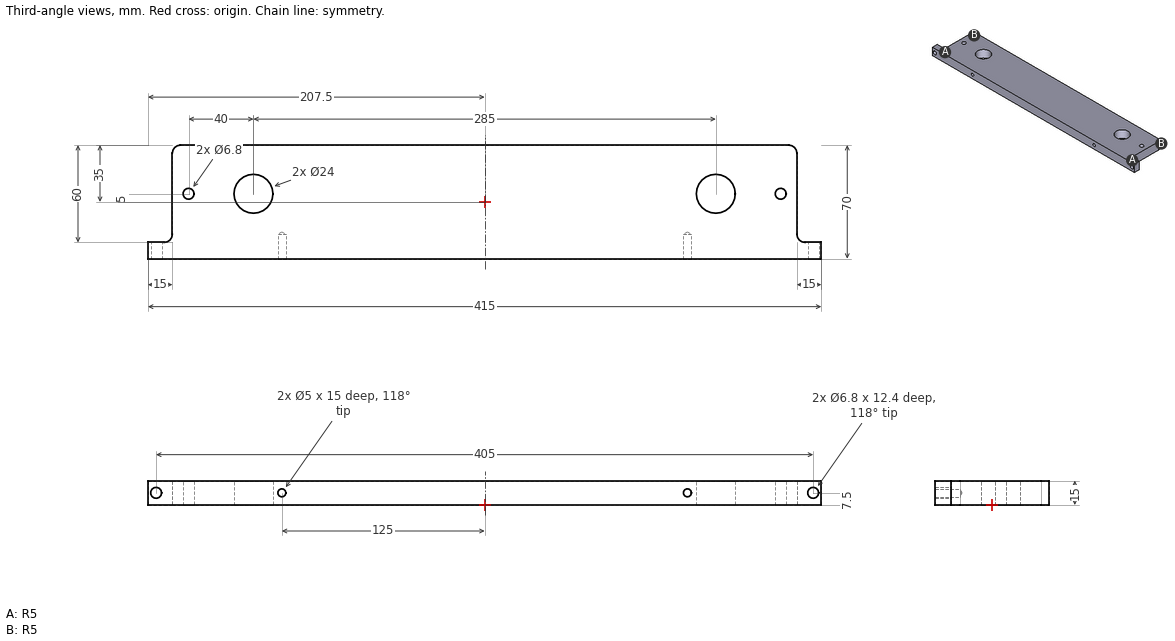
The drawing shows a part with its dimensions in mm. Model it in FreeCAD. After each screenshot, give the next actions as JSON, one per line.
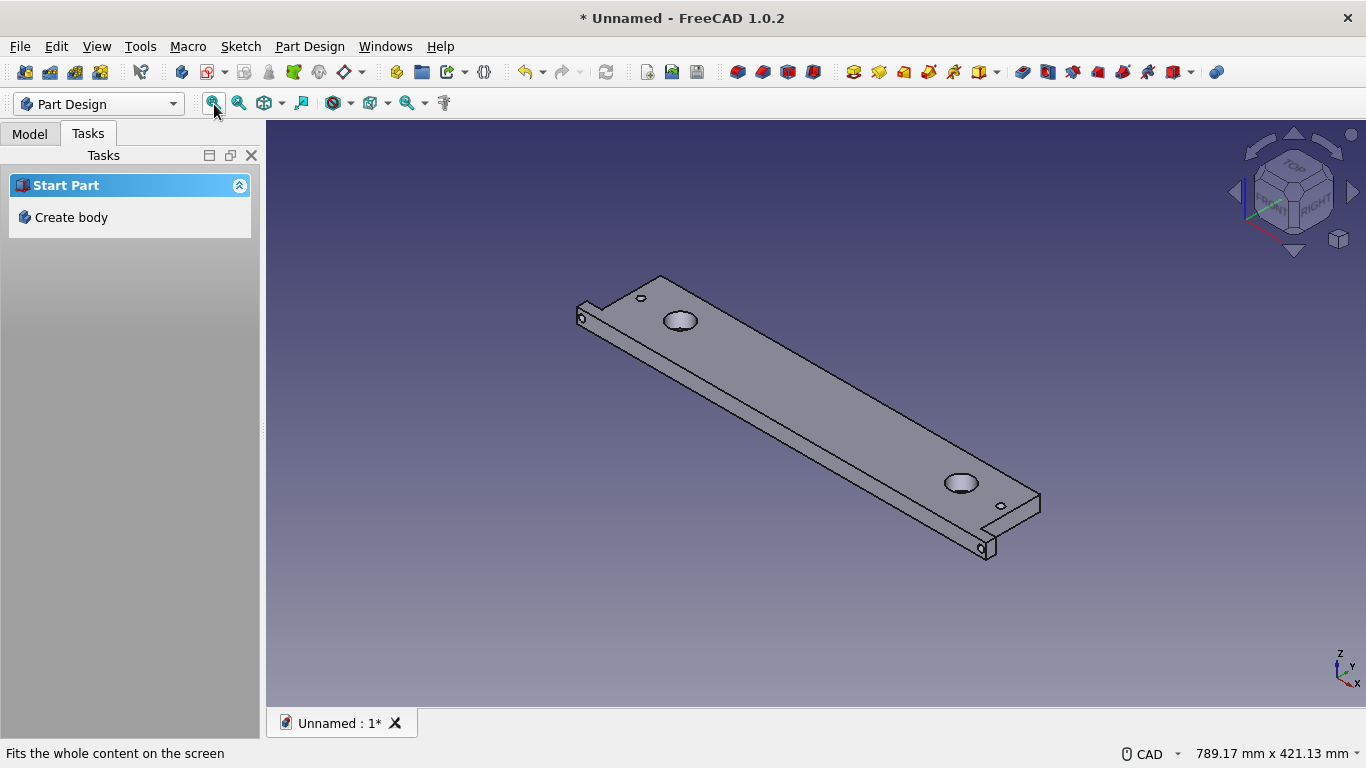
{"action": "scroll", "coordinate": [602, 317], "scroll_direction": "up", "scroll_amount": 4}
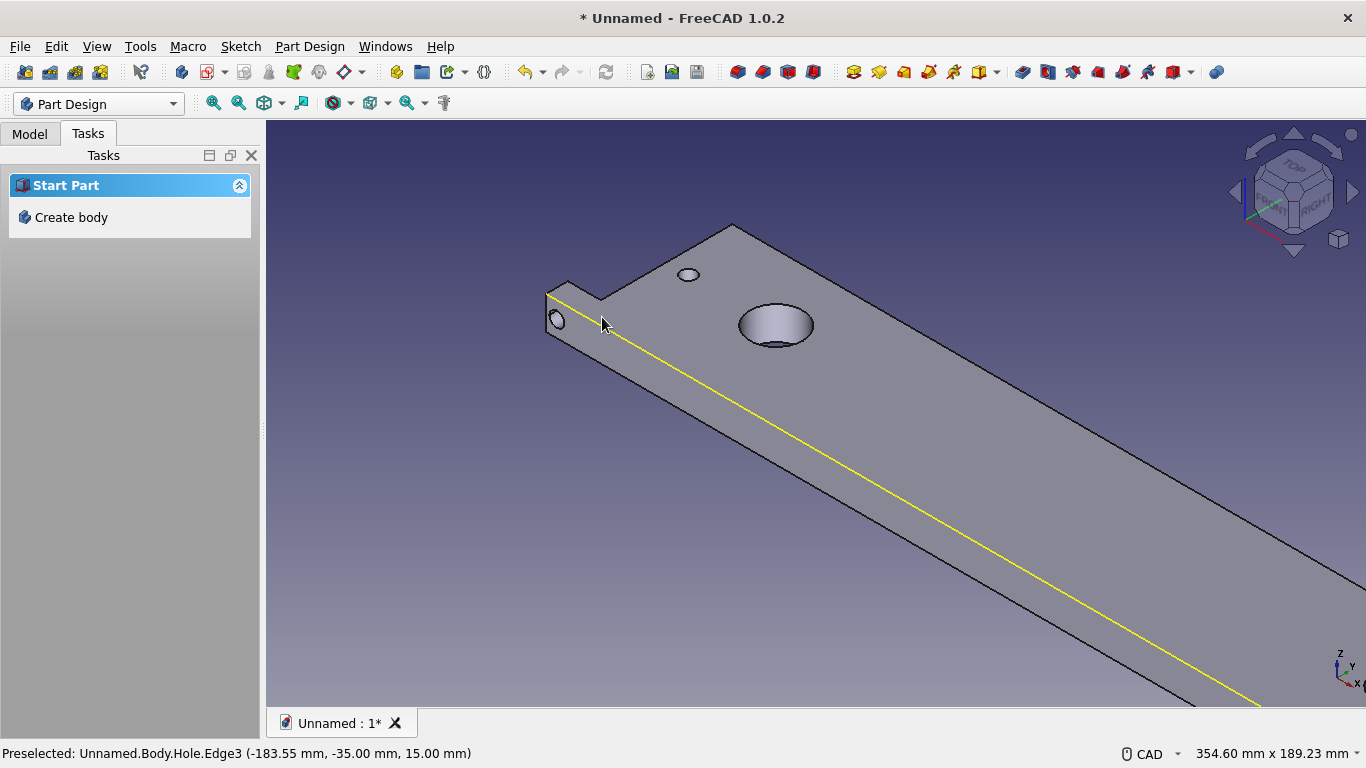
{"action": "key", "text": "v f"}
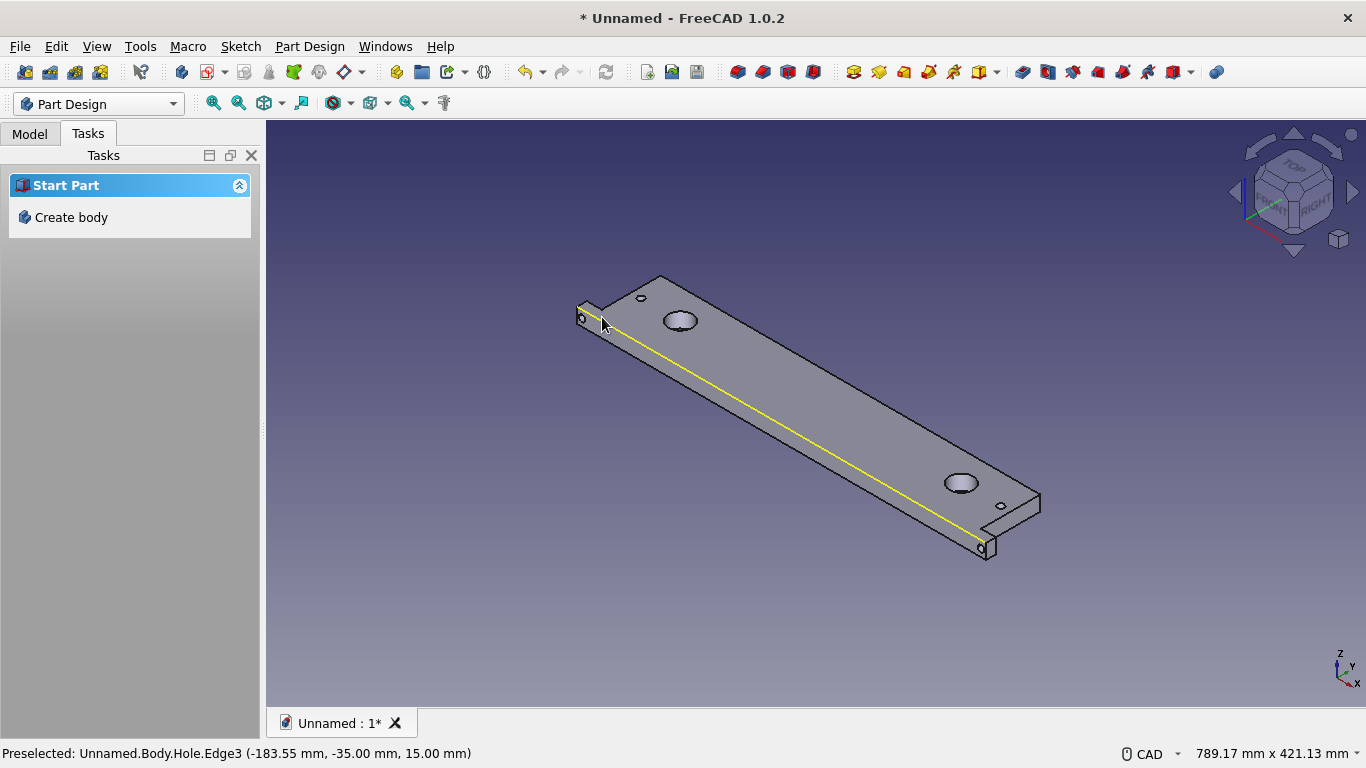
{"action": "key", "text": "2"}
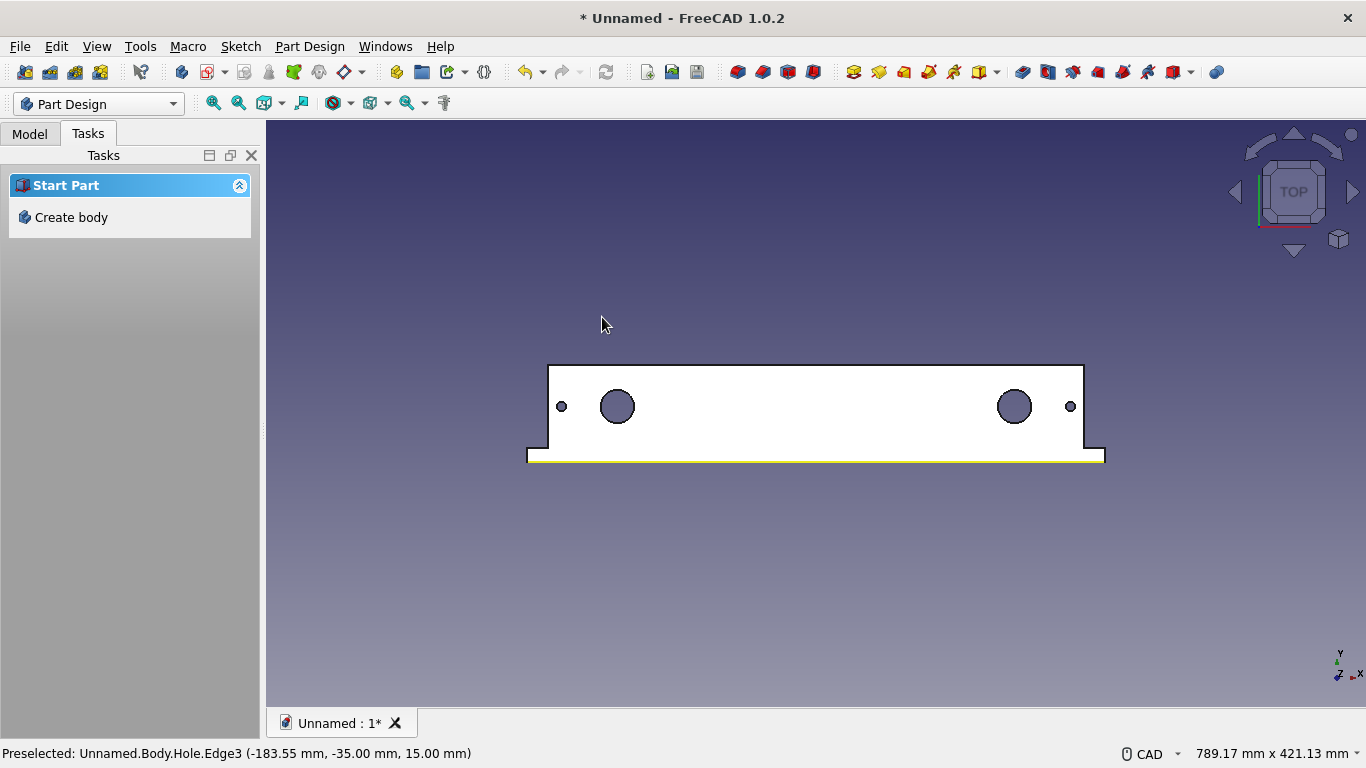
{"action": "scroll", "coordinate": [548, 447], "scroll_direction": "up", "scroll_amount": 4}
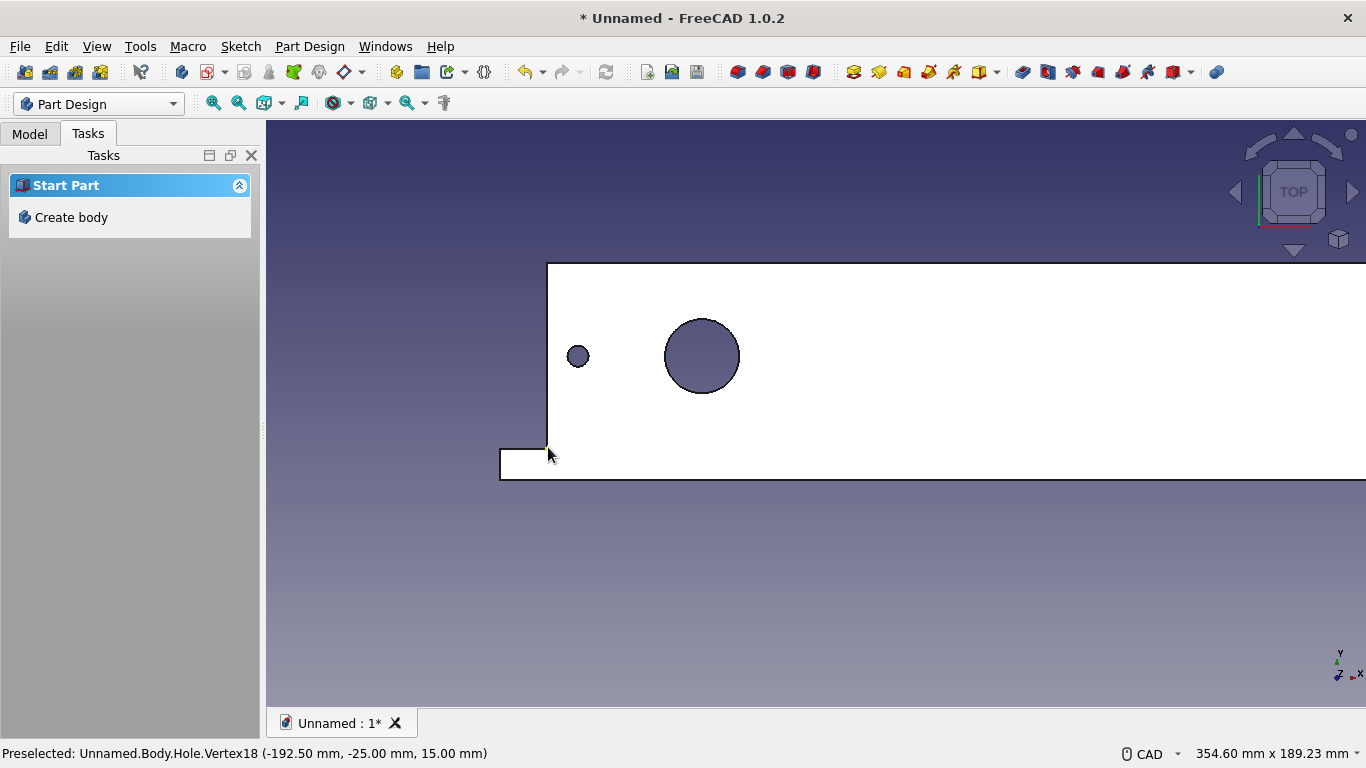
{"action": "key", "text": "v f"}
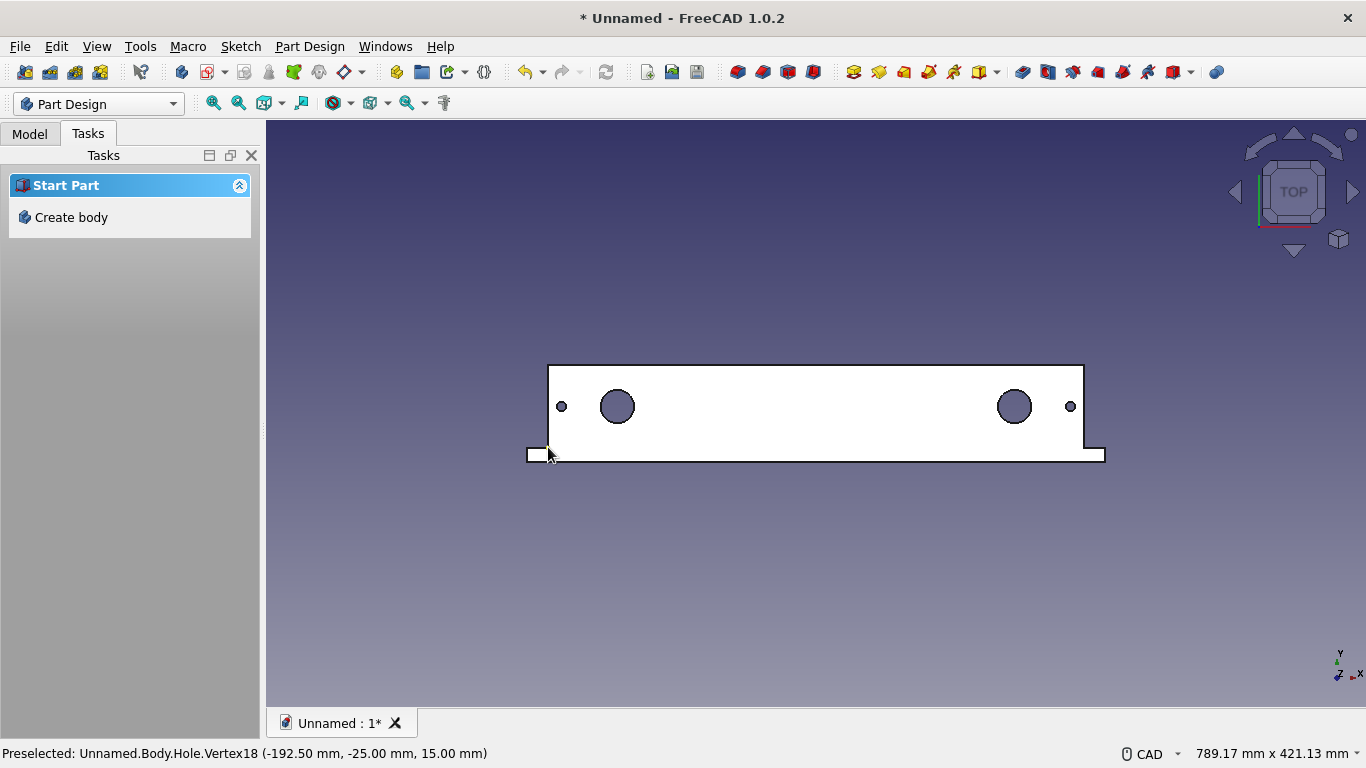
{"action": "key", "text": "1"}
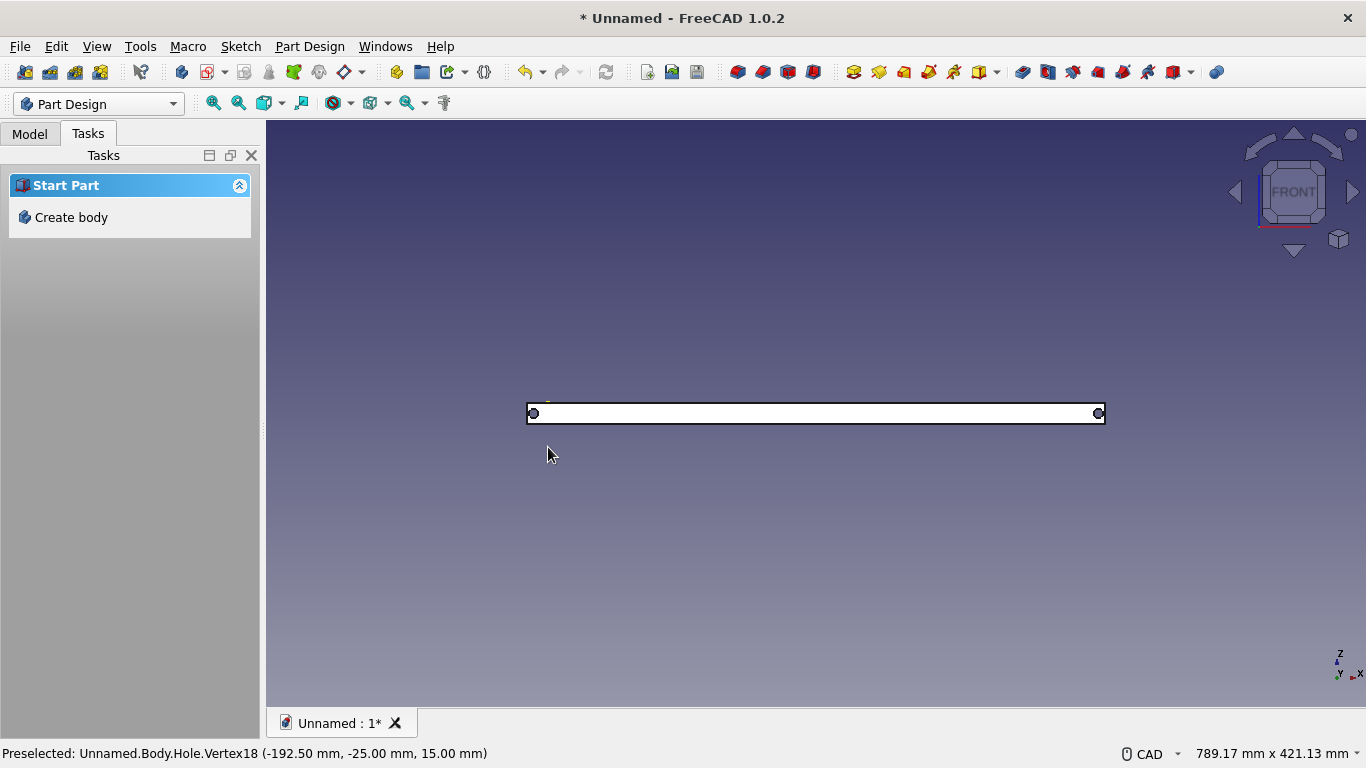
{"action": "scroll", "coordinate": [548, 412], "scroll_direction": "up", "scroll_amount": 4}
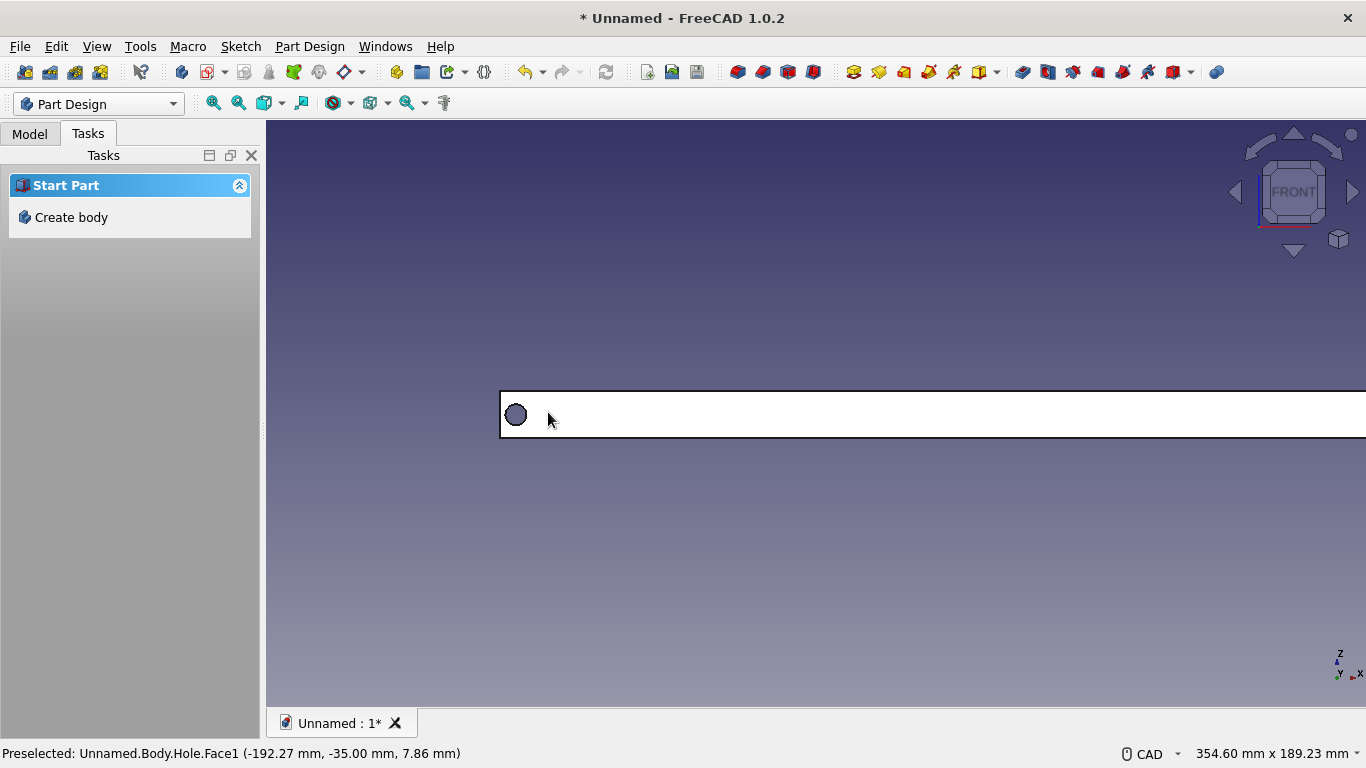
{"action": "key", "text": "v f"}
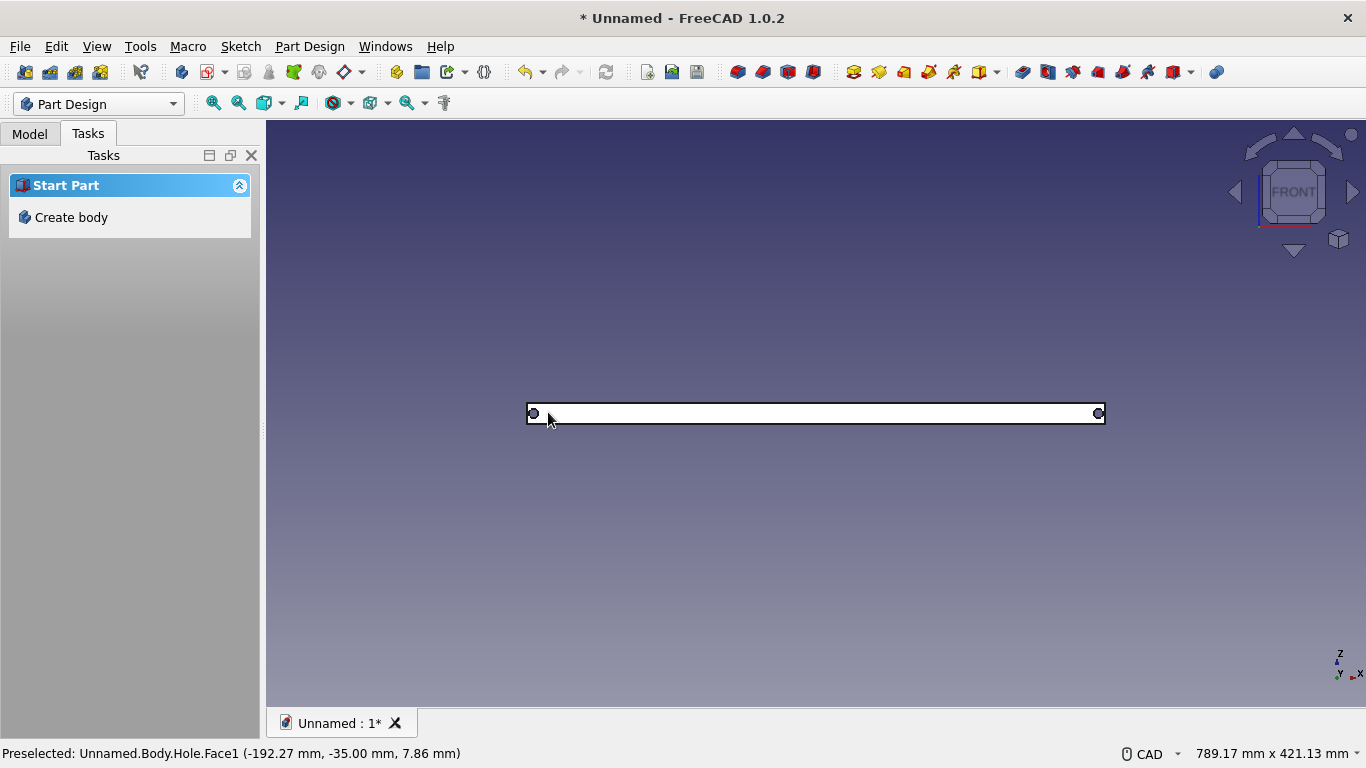
{"action": "key", "text": "3"}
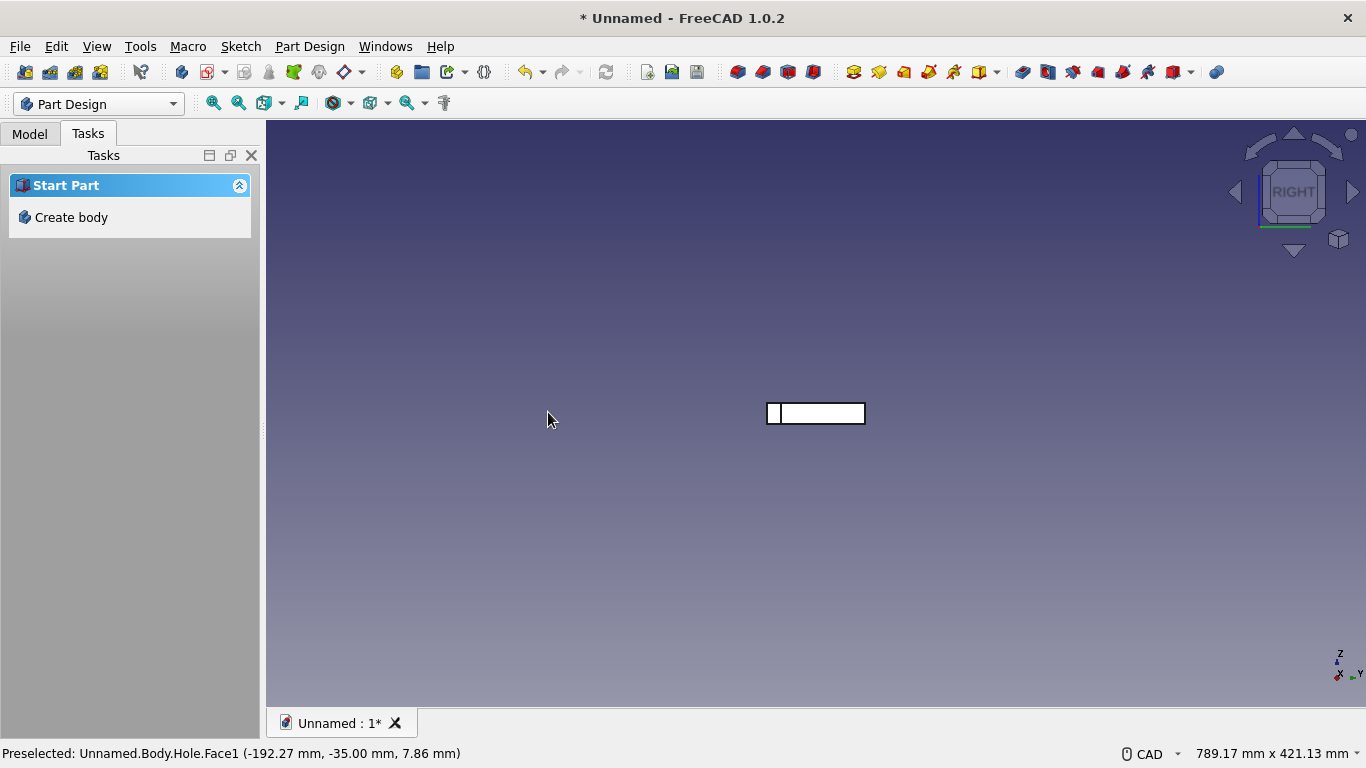
{"action": "key", "text": "v f"}